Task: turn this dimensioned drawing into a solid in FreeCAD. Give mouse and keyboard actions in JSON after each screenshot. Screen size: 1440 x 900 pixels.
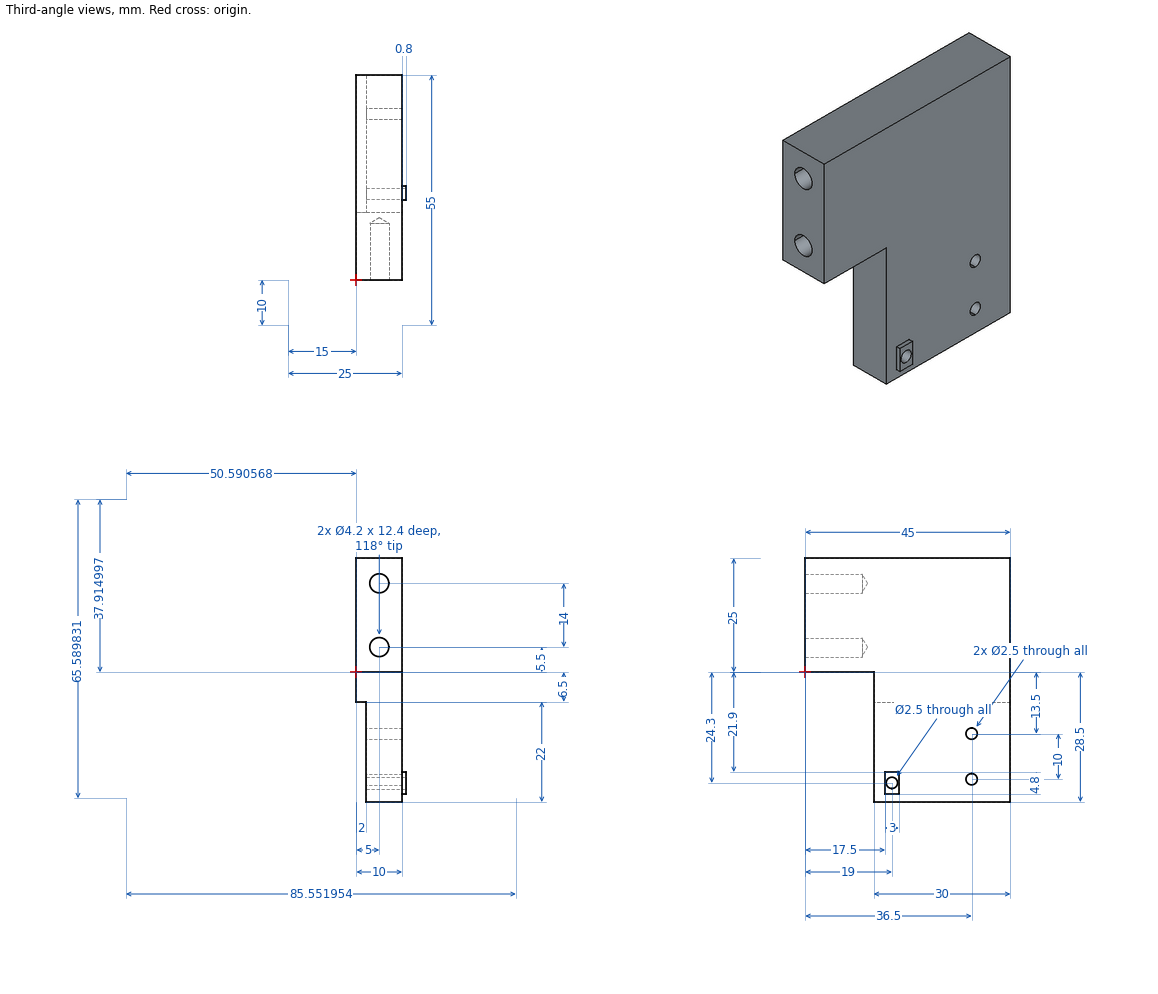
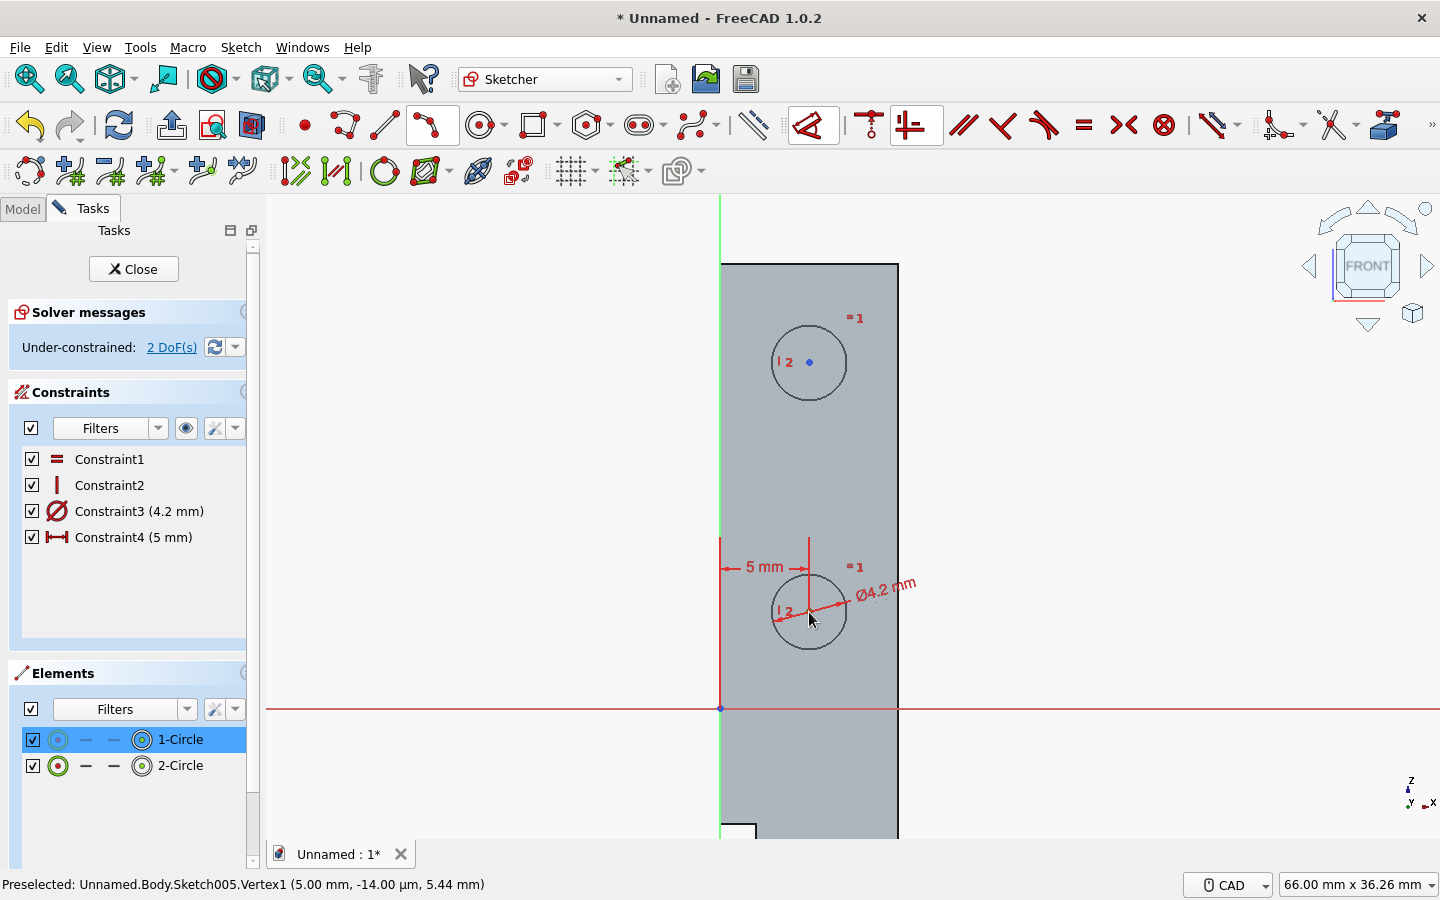
{"action": "key", "text": "i"}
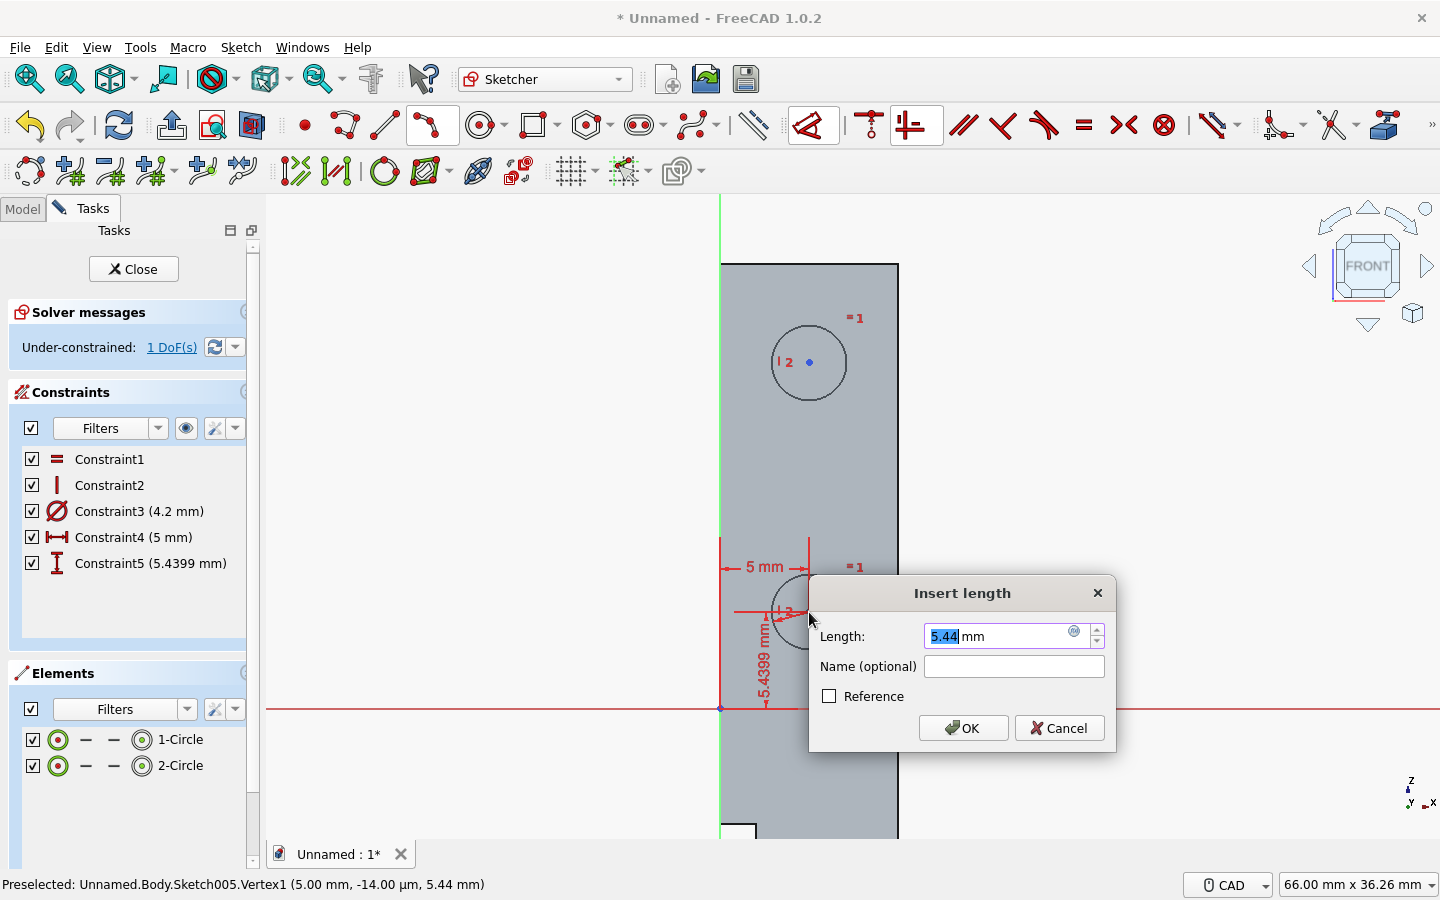
{"action": "type", "text": "5.5"}
{"action": "key", "text": "Return"}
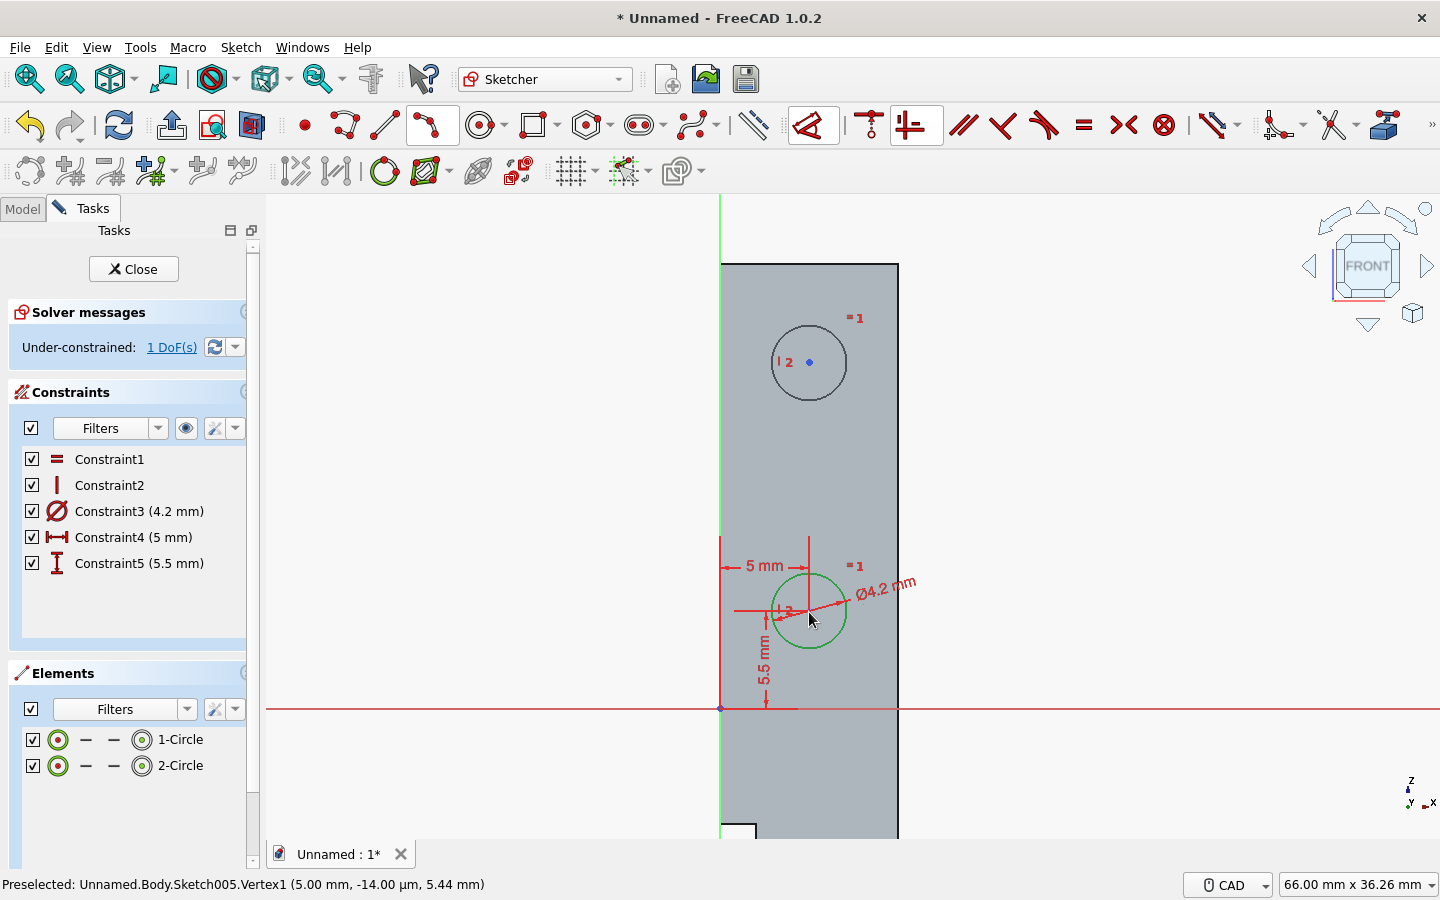
{"action": "left_click", "coordinate": [809, 611]}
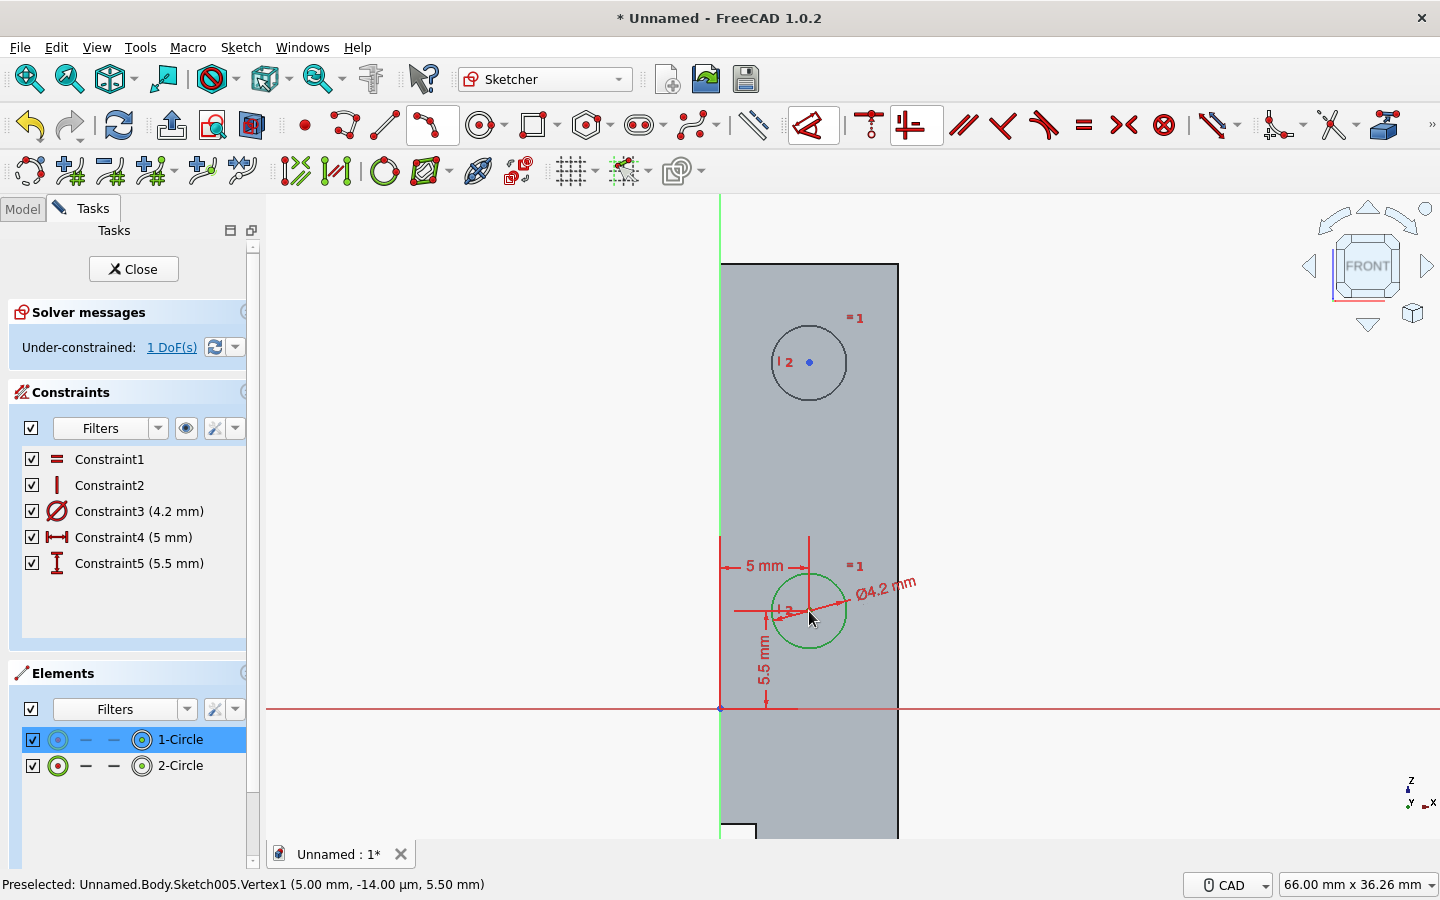
{"action": "left_click", "coordinate": [809, 363]}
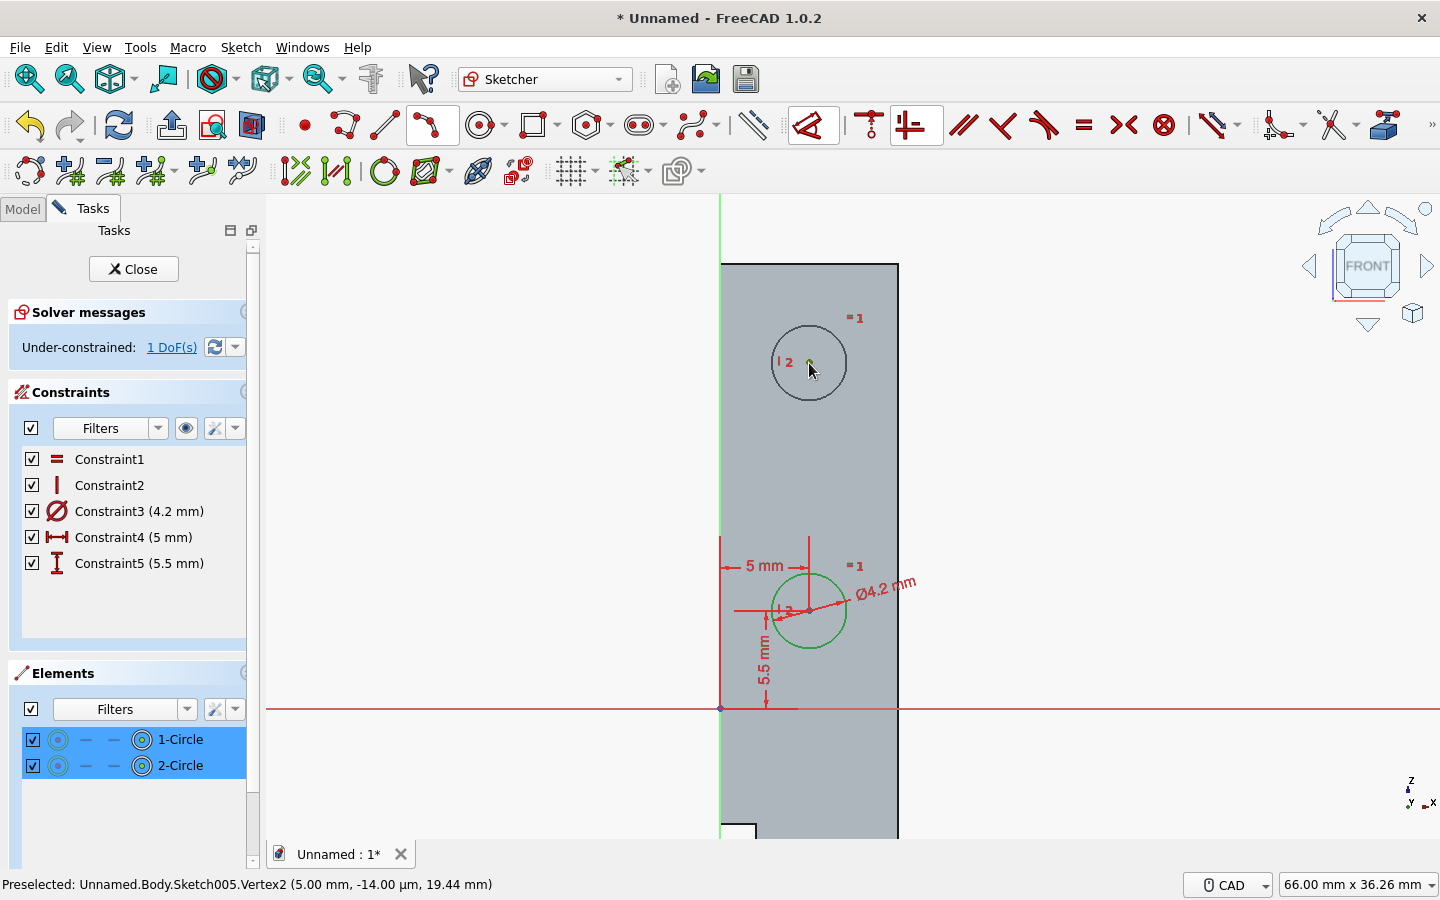
{"action": "key", "text": "i"}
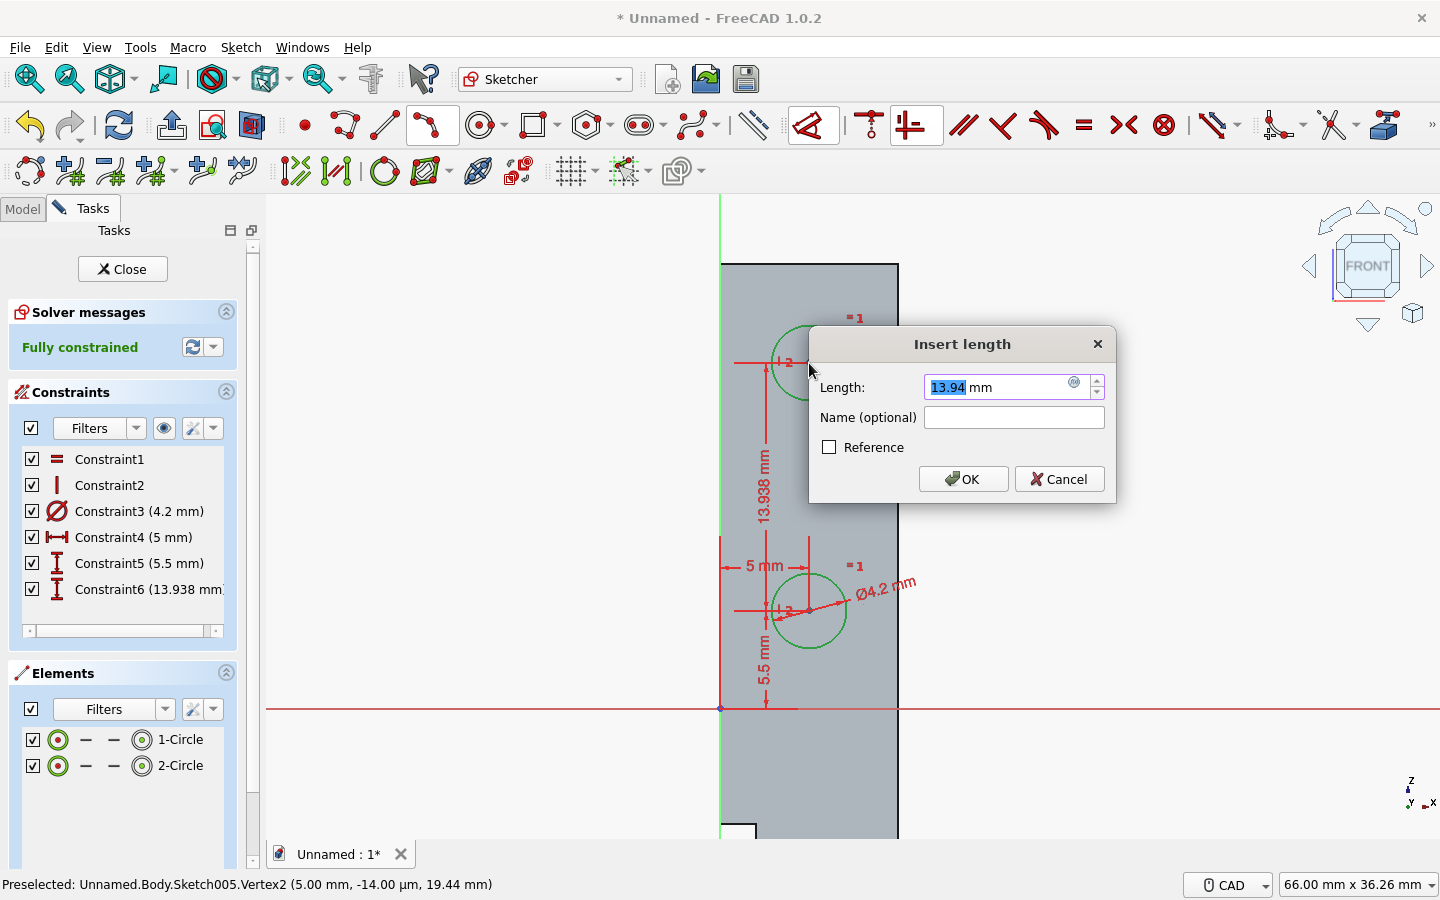
{"action": "type", "text": "14"}
{"action": "key", "text": "Return"}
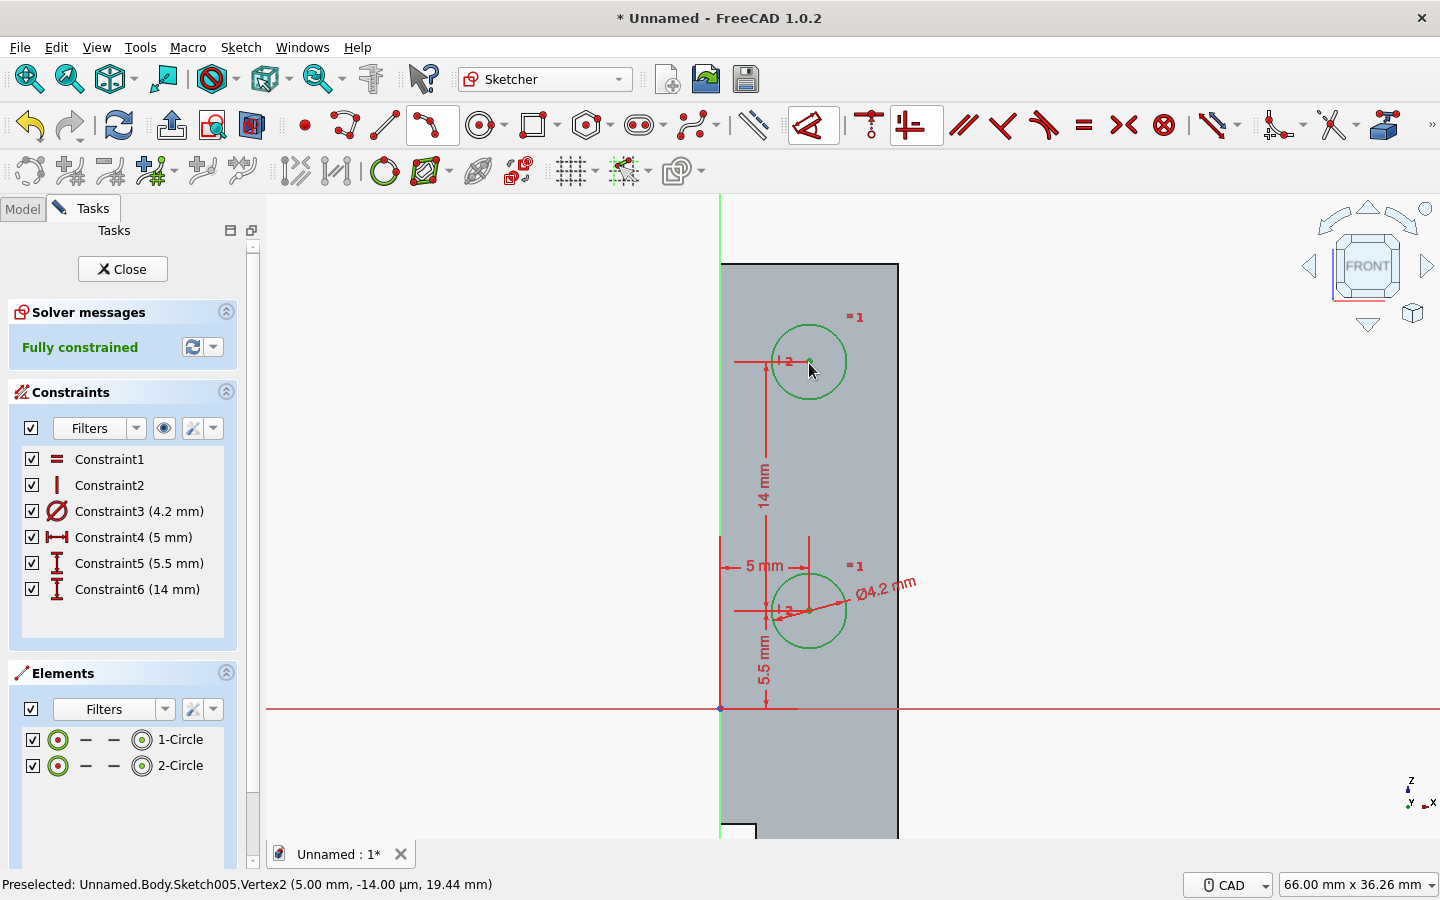
{"action": "left_click", "coordinate": [123, 269]}